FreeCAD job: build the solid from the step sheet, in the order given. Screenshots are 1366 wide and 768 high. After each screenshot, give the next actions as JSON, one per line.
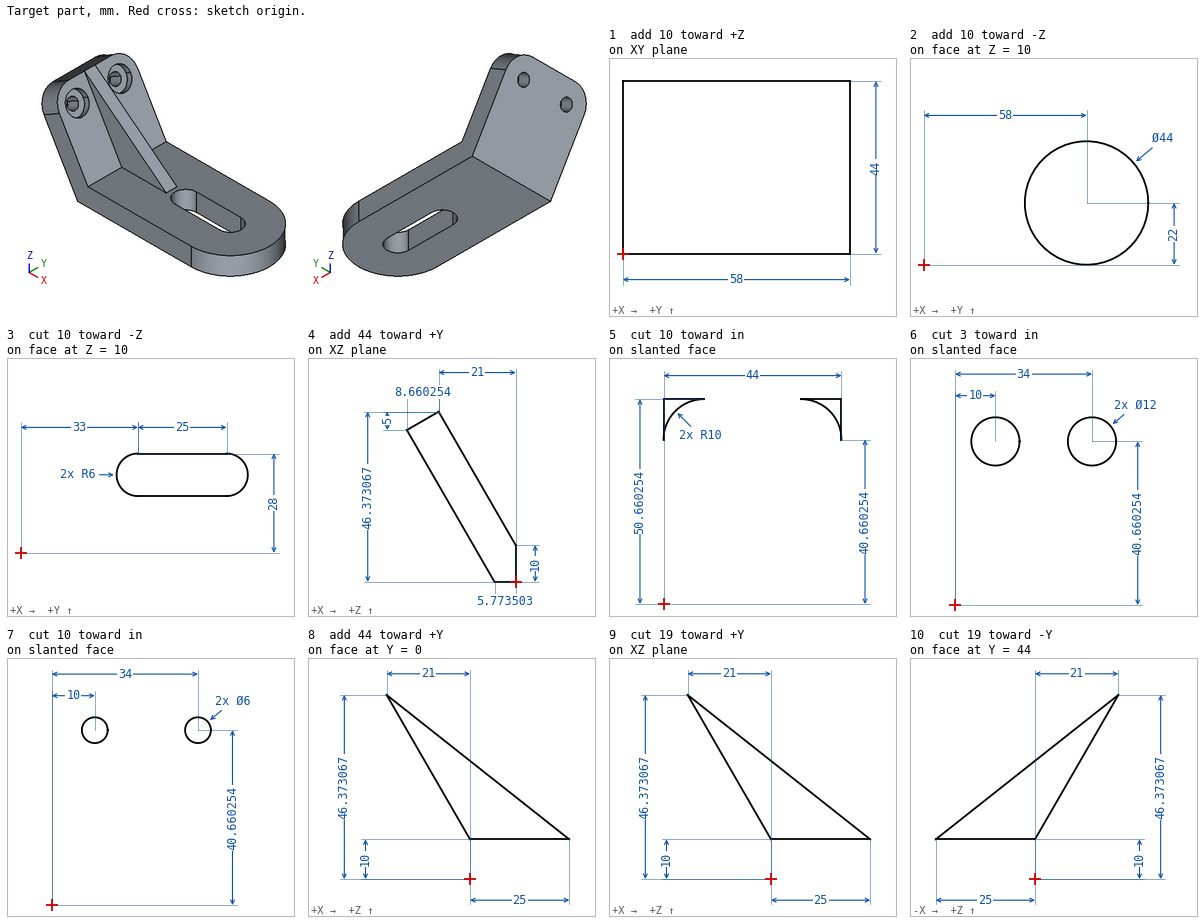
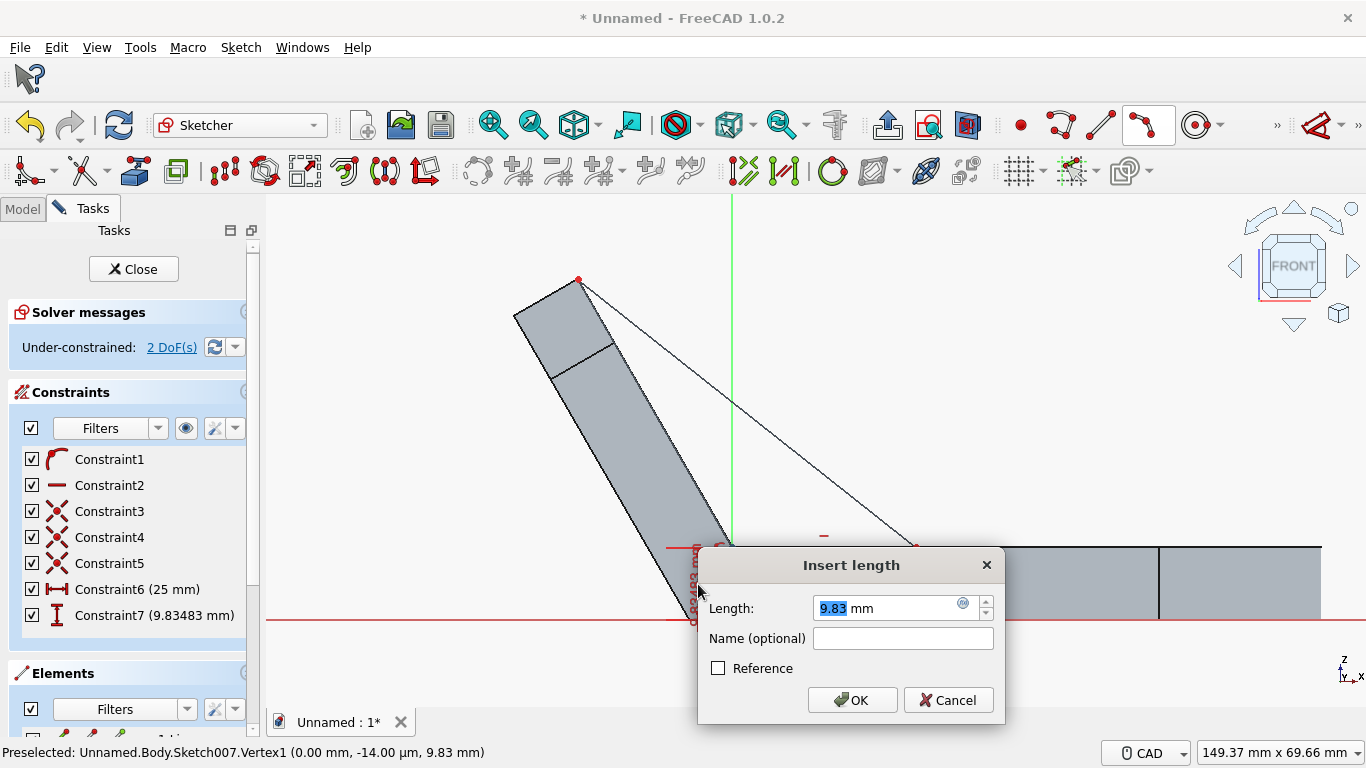
{"action": "type", "text": "10"}
{"action": "key", "text": "Return"}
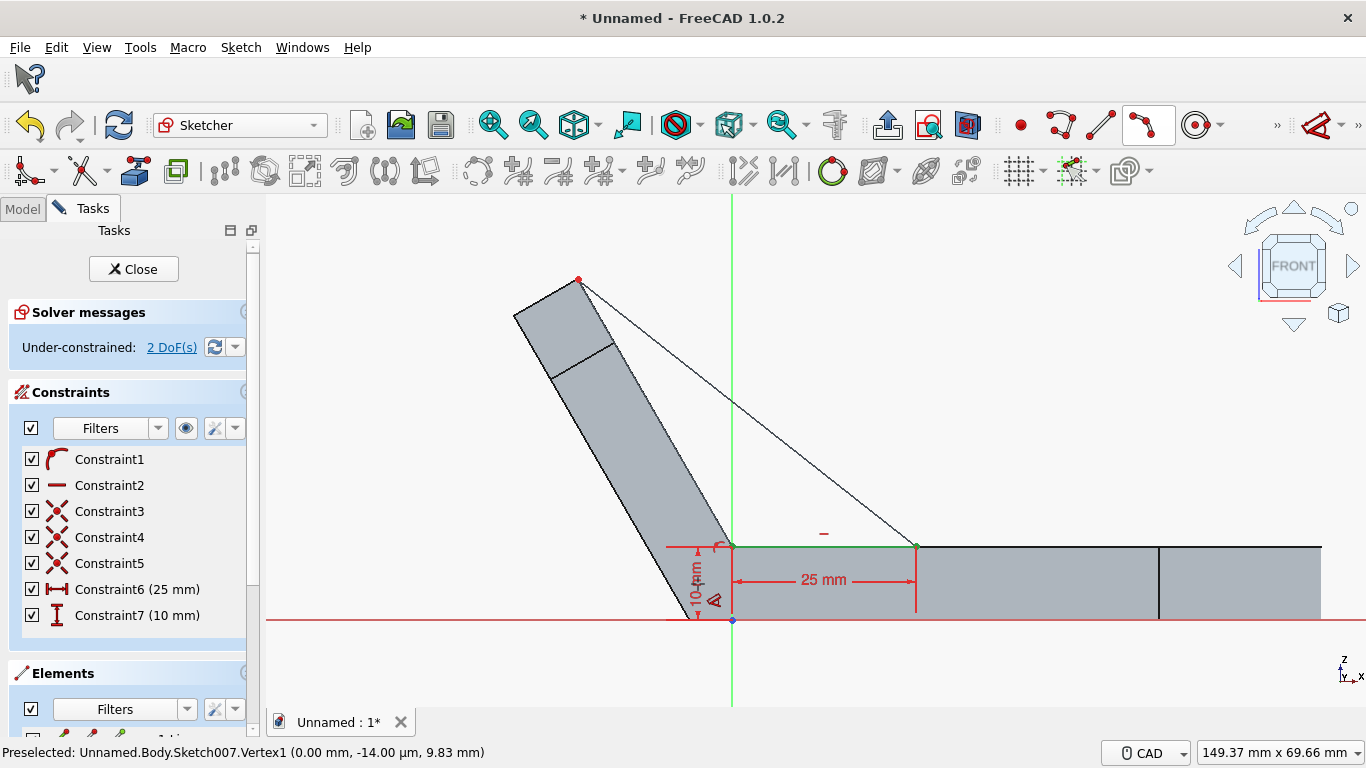
{"action": "left_click", "coordinate": [578, 280]}
{"action": "left_click", "coordinate": [655, 654]}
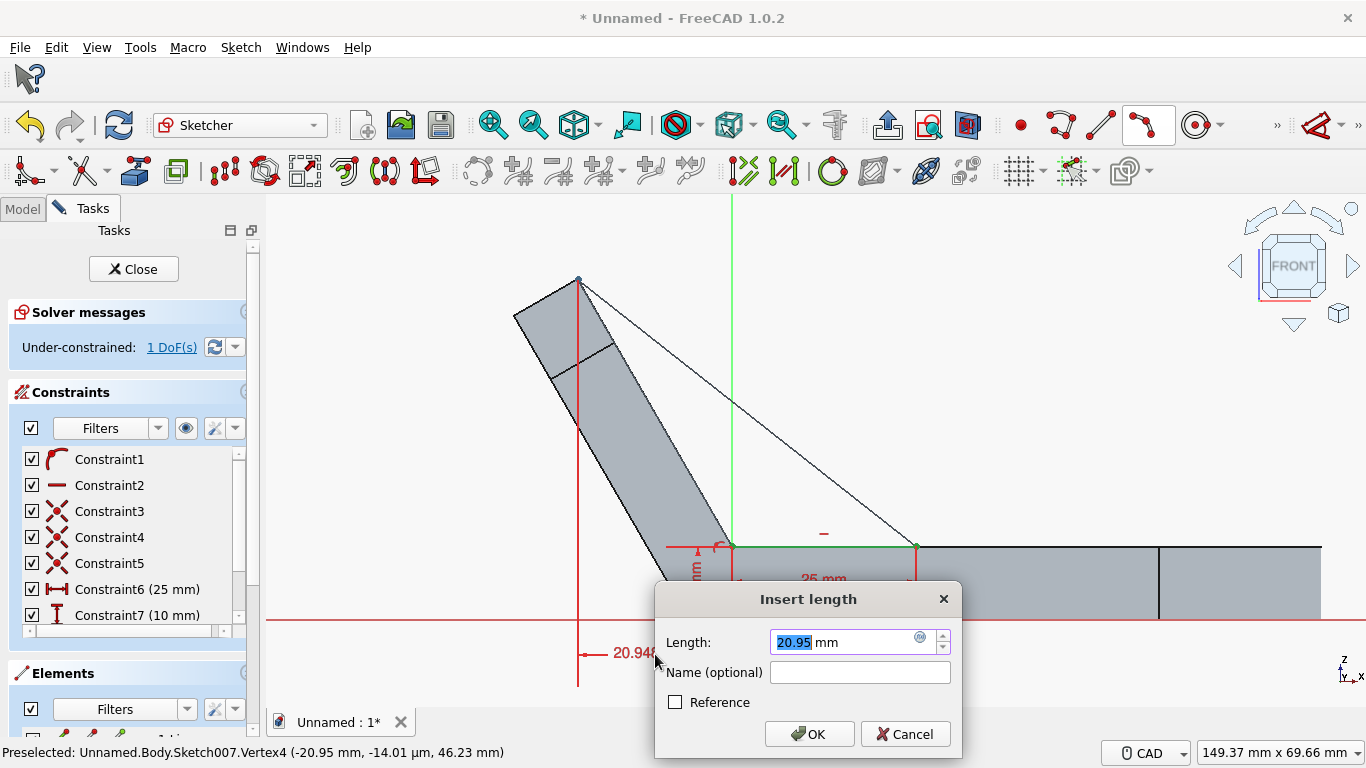
{"action": "type", "text": "21"}
{"action": "key", "text": "Return"}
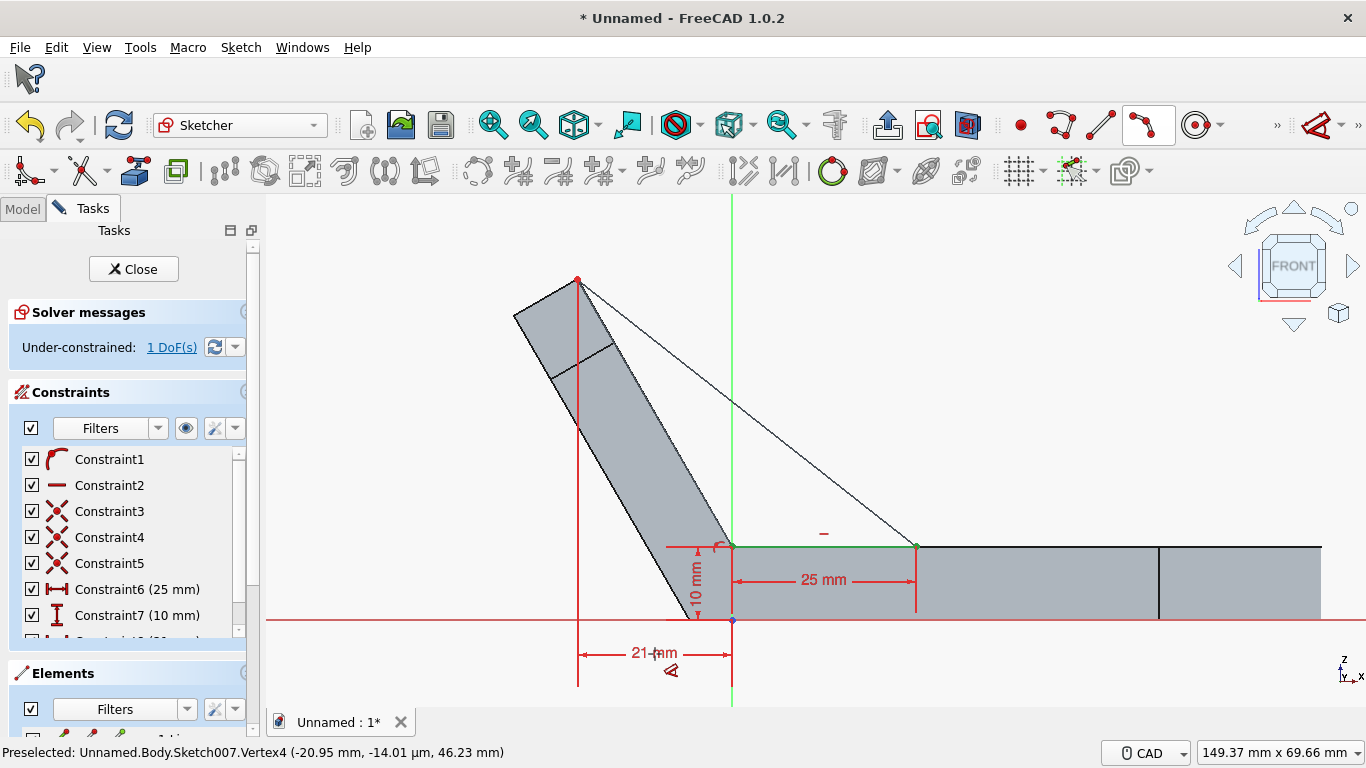
{"action": "left_click", "coordinate": [578, 280]}
{"action": "left_click", "coordinate": [544, 450]}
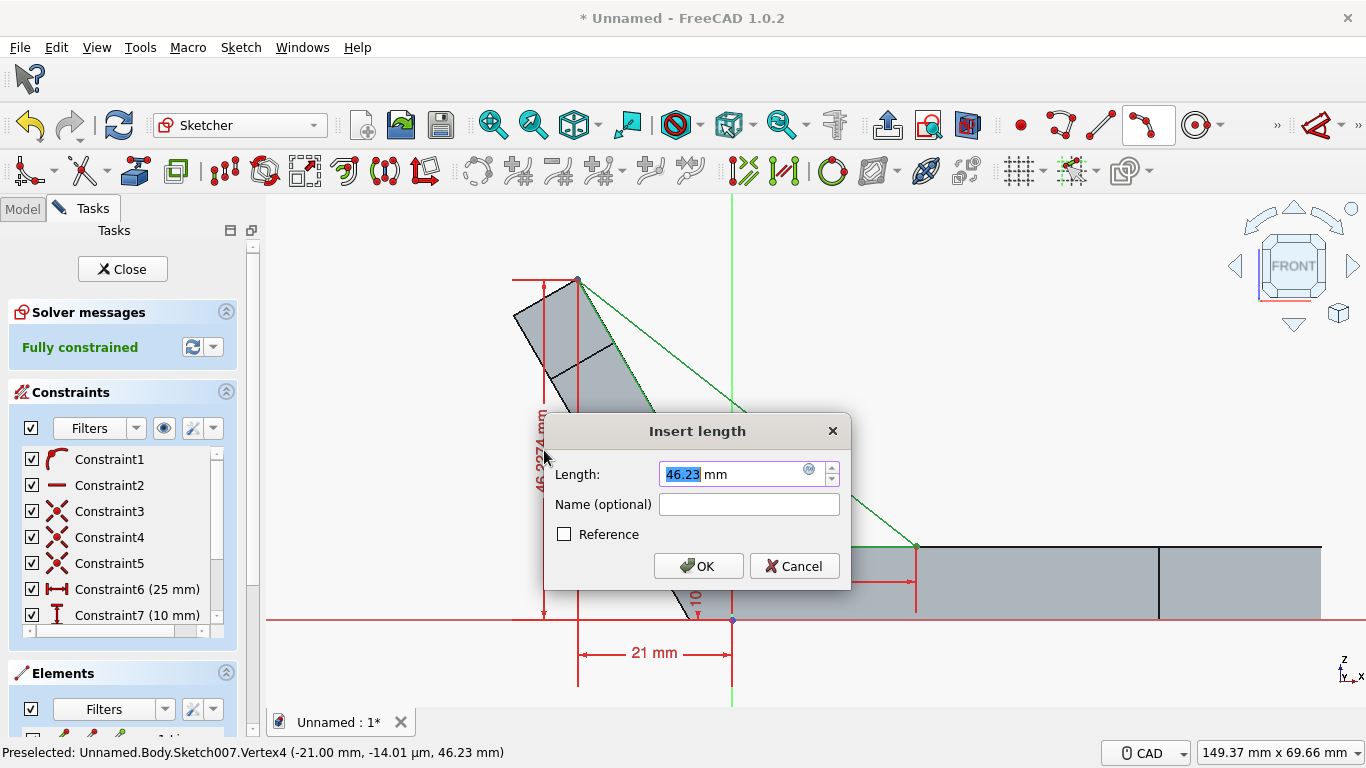
{"action": "type", "text": "46.373067"}
{"action": "key", "text": "Return"}
{"action": "key", "text": "Escape"}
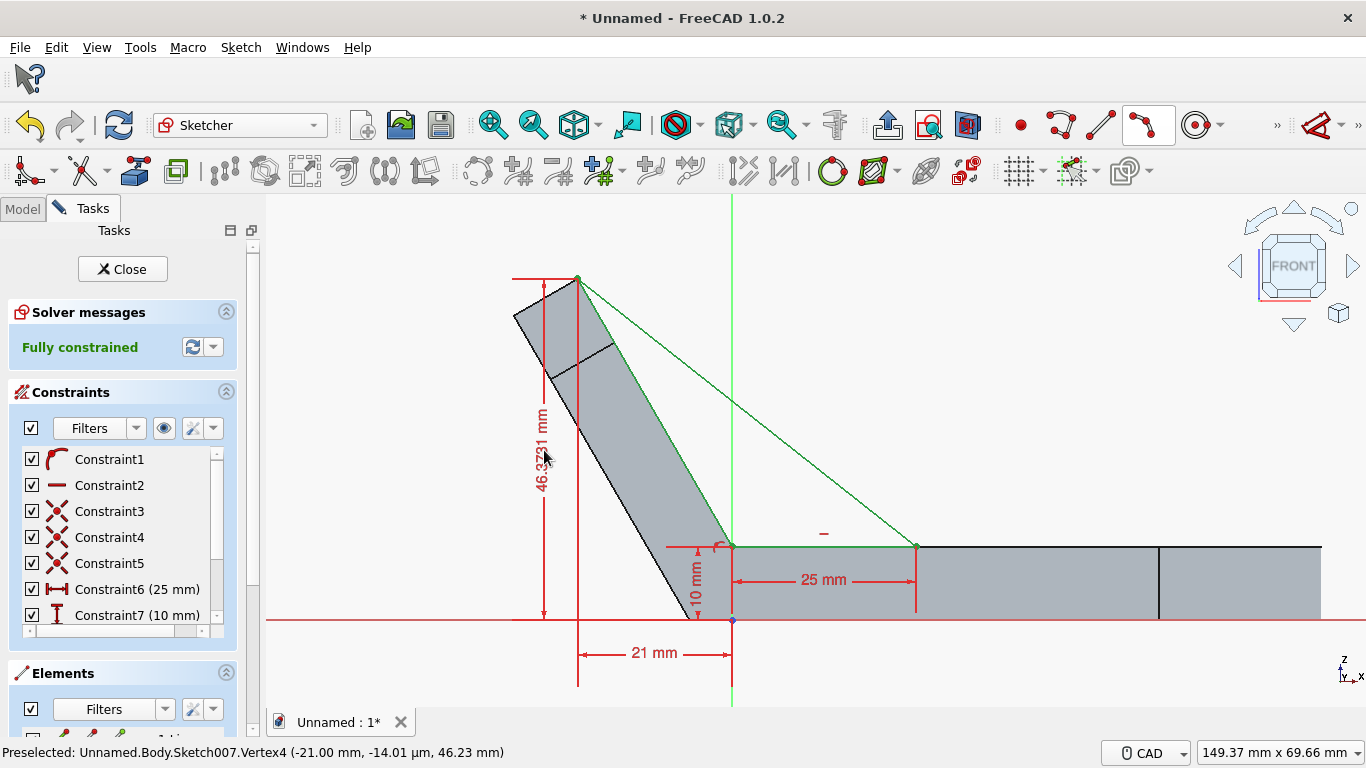
{"action": "left_click", "coordinate": [123, 269]}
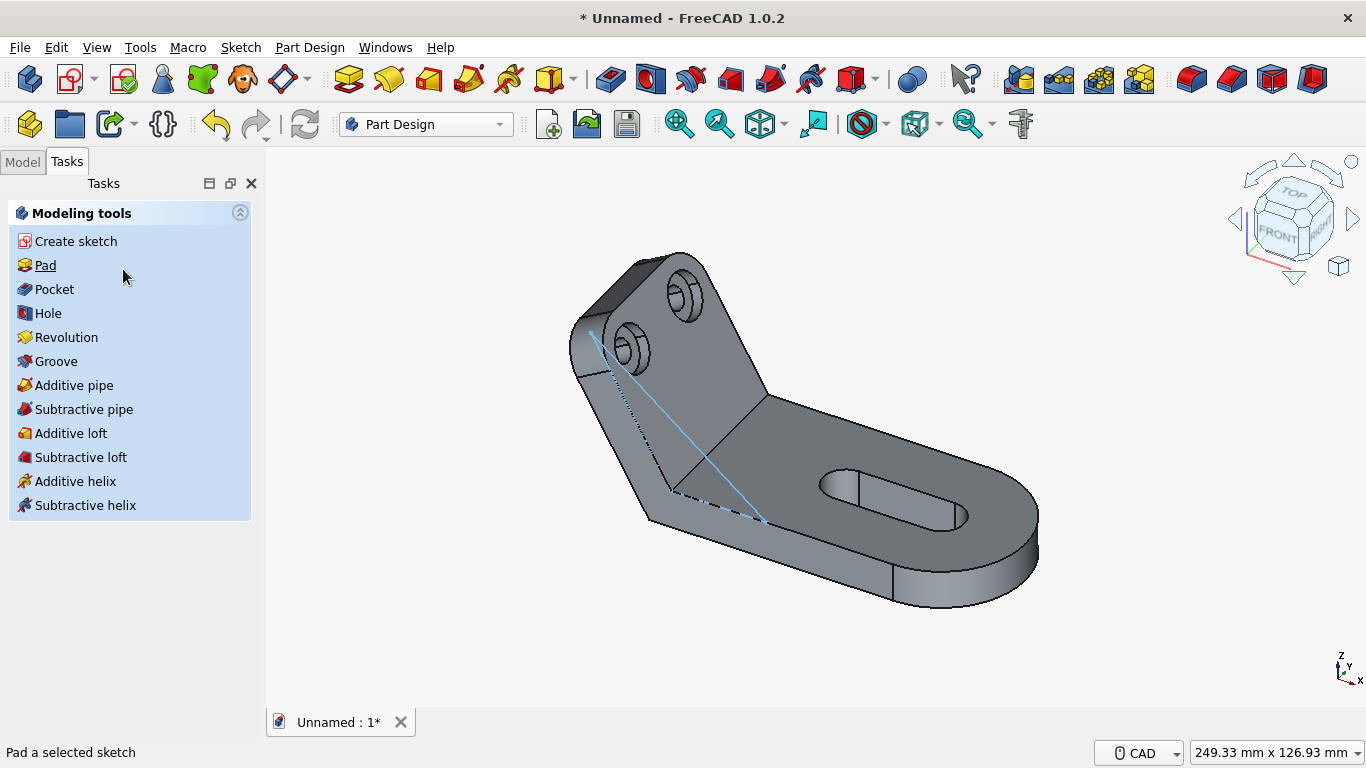
{"action": "left_click", "coordinate": [350, 80]}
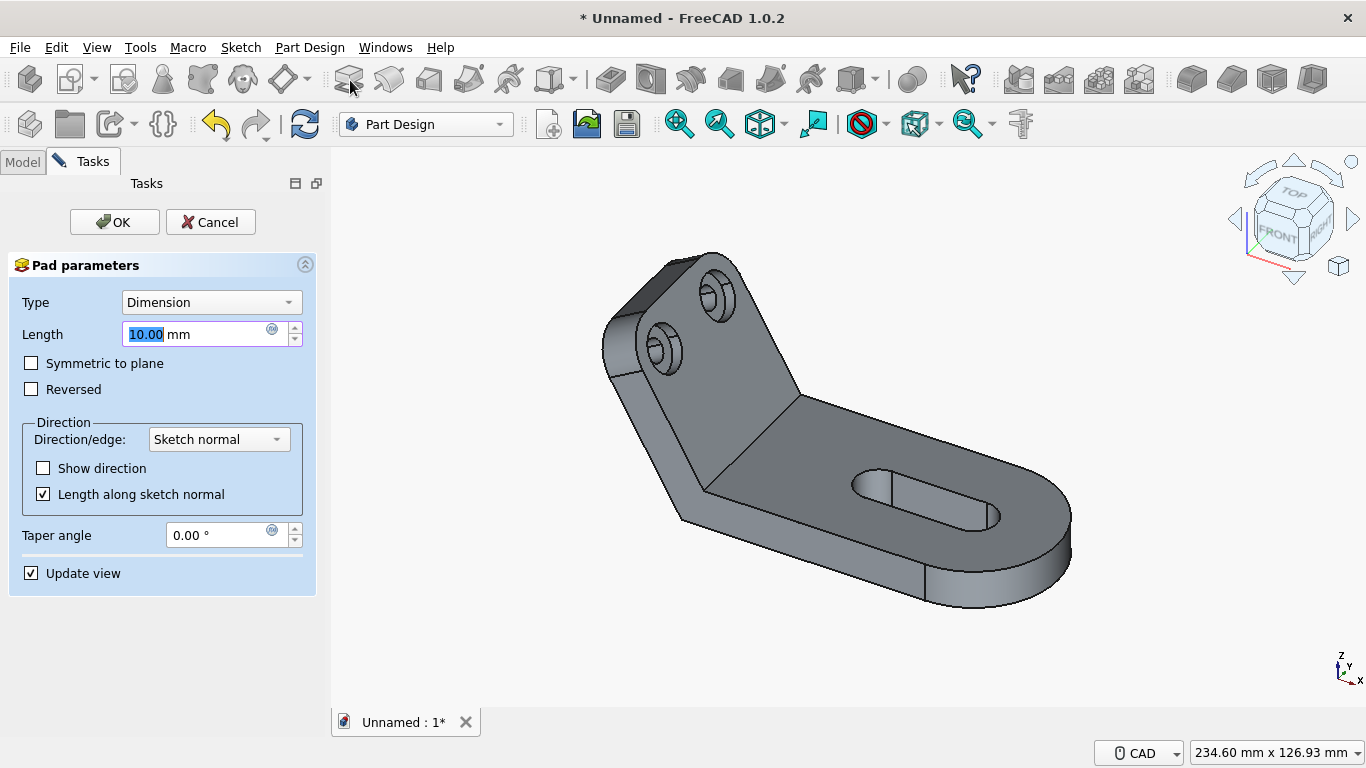
{"action": "type", "text": "44"}
{"action": "key", "text": "Tab"}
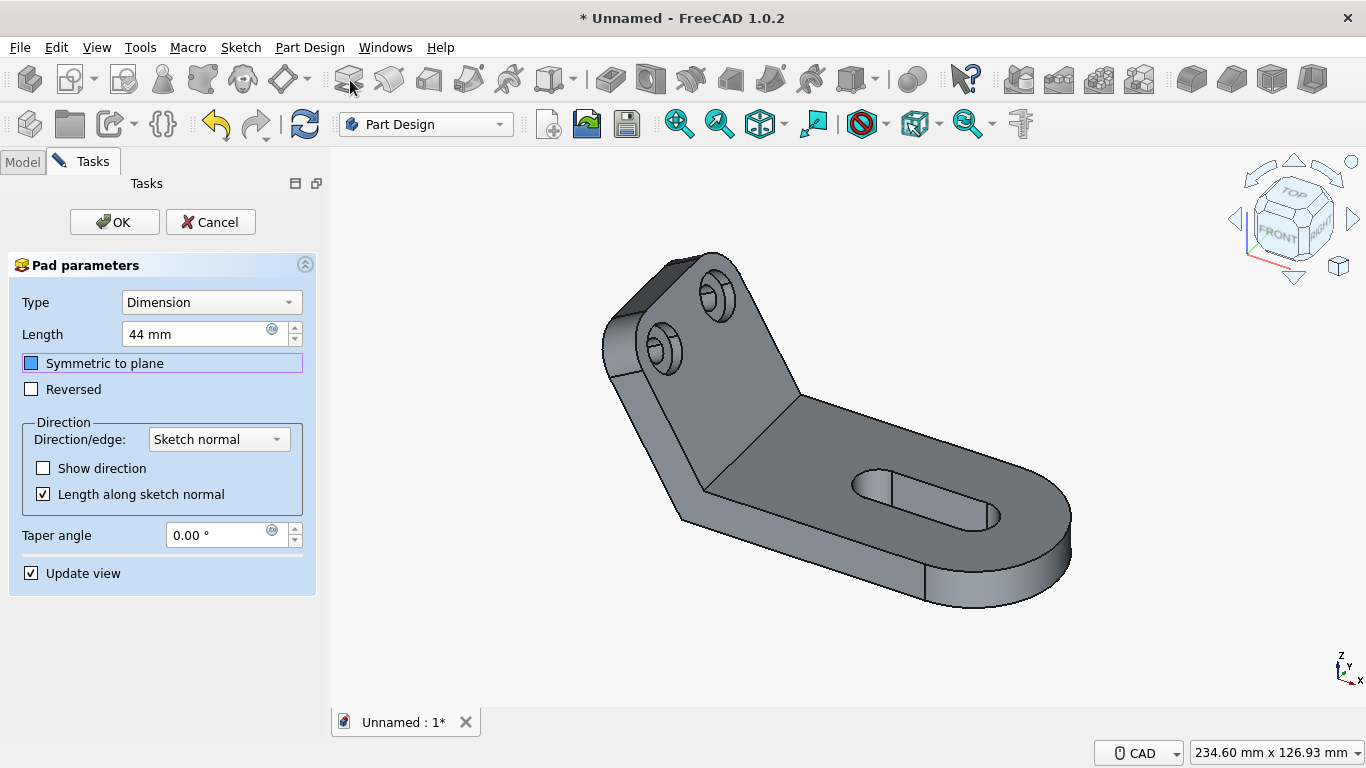
{"action": "left_click", "coordinate": [30, 389]}